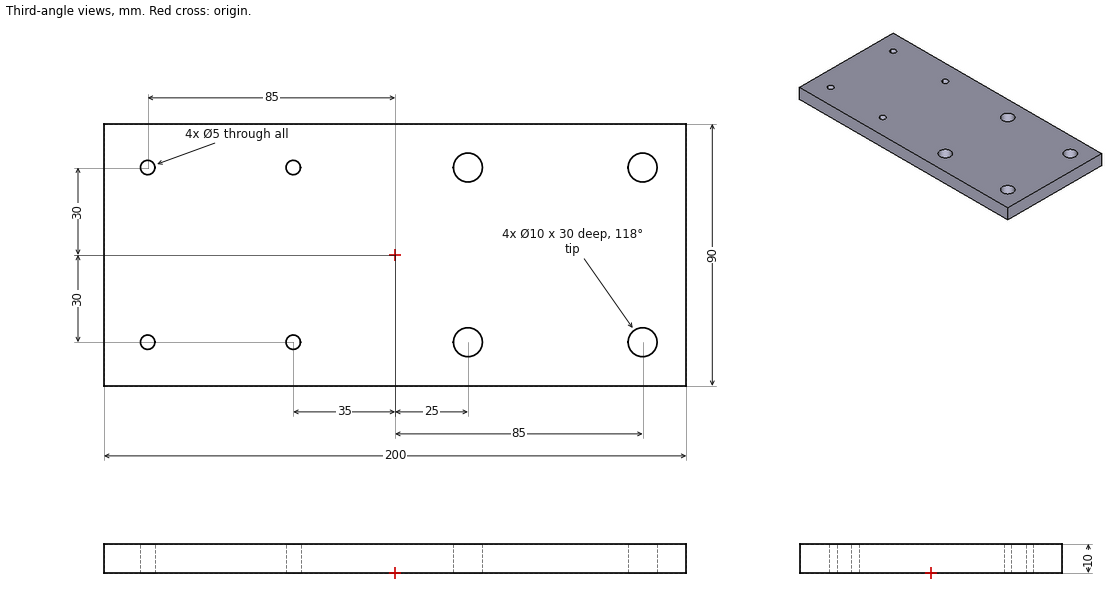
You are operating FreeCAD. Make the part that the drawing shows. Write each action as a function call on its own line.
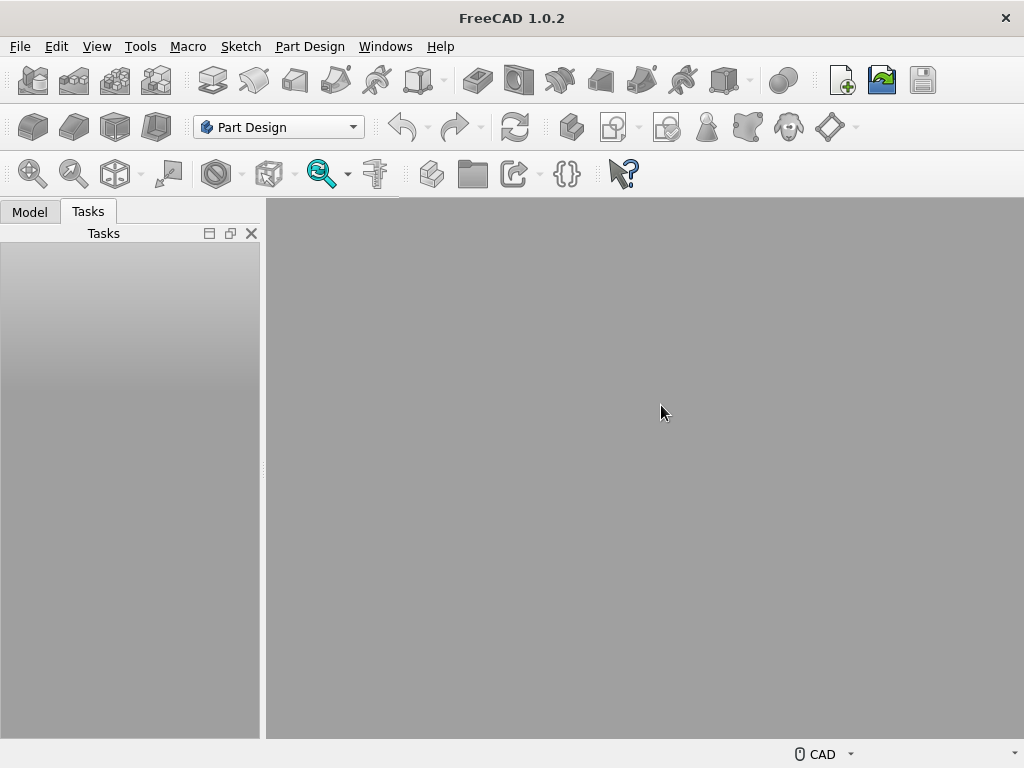
key(ctrl+n)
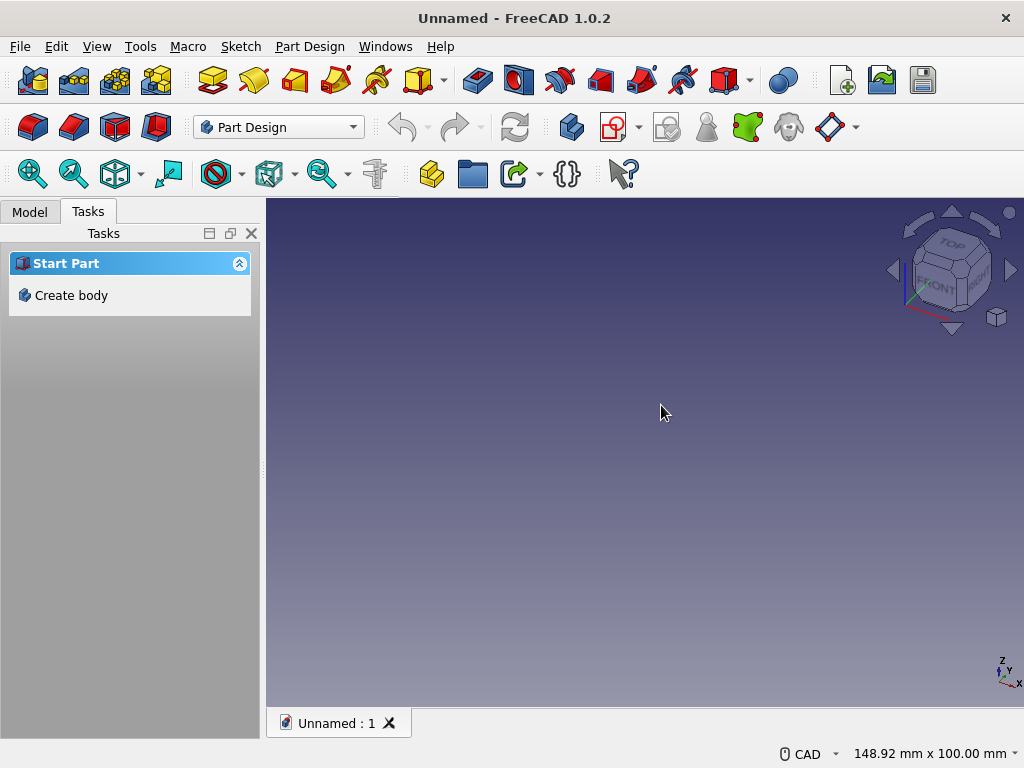
click(612, 128)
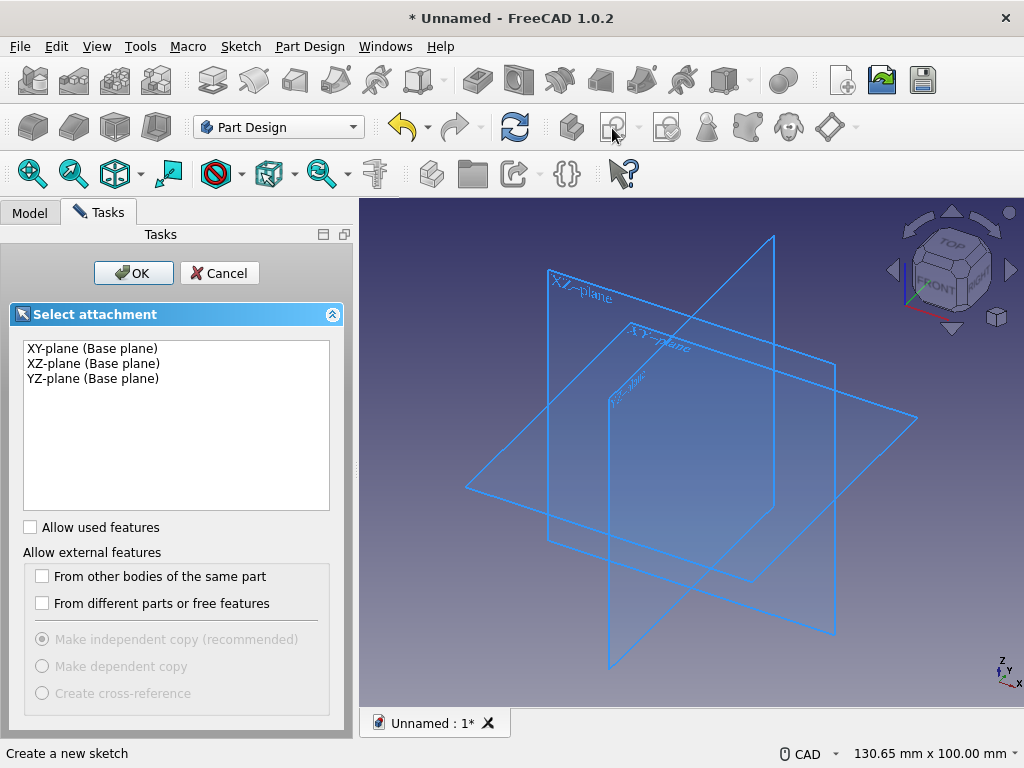
click(84, 348)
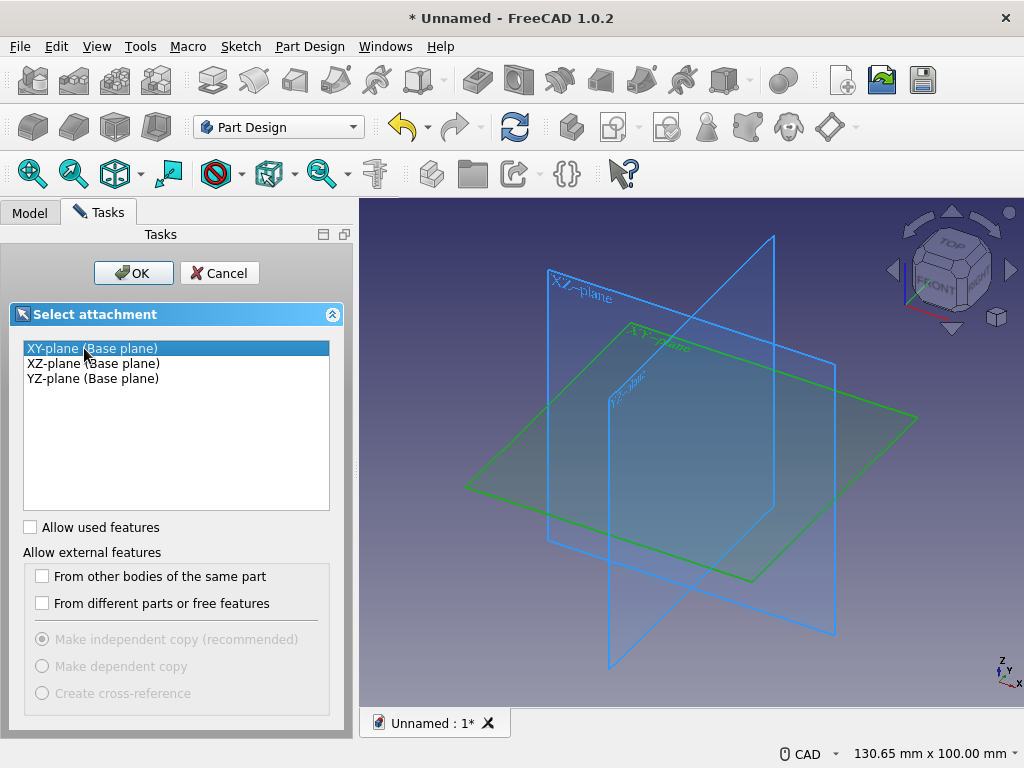
click(134, 273)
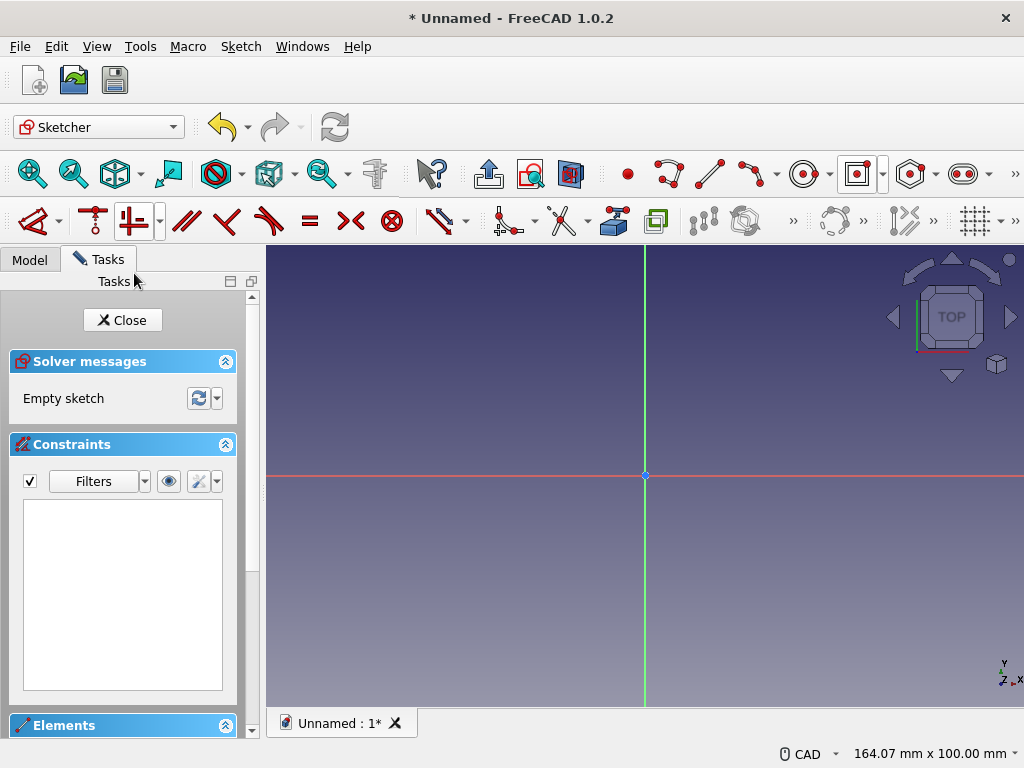
scroll(521, 476, down, 4)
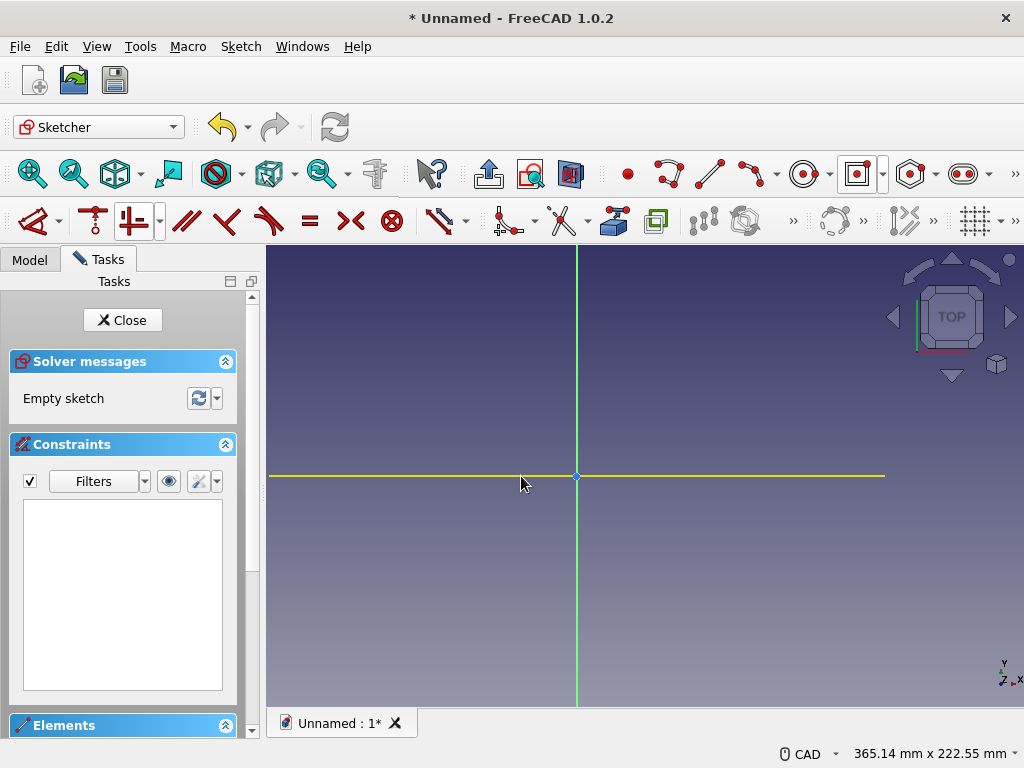
click(856, 174)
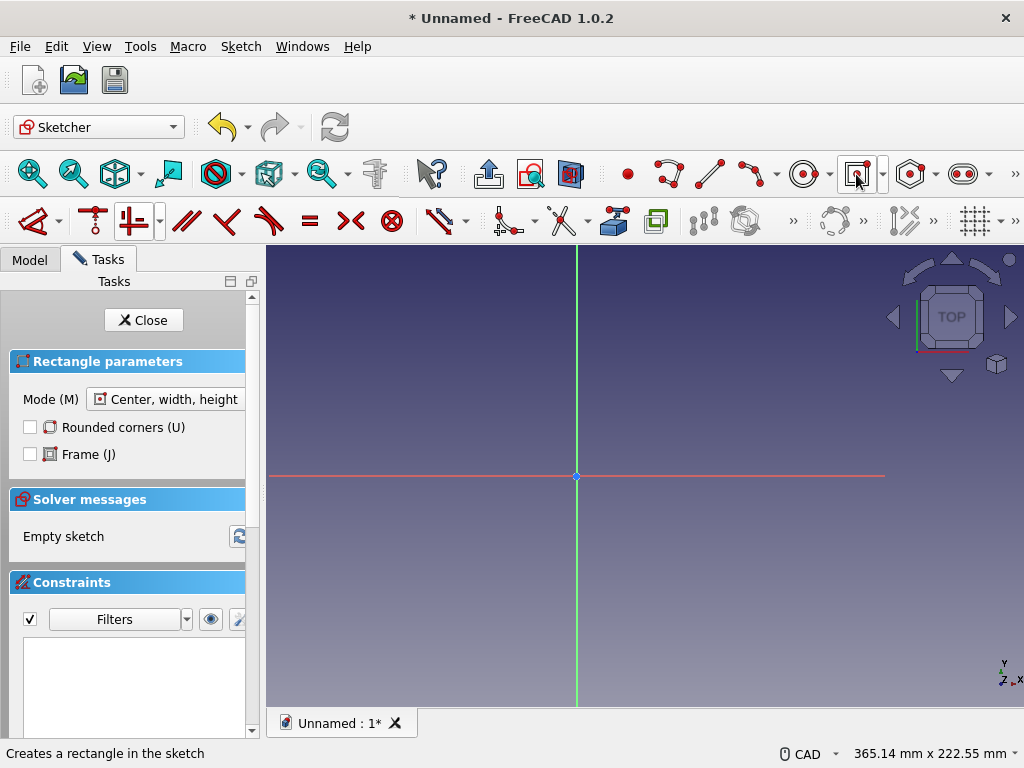
click(577, 476)
move(784, 383)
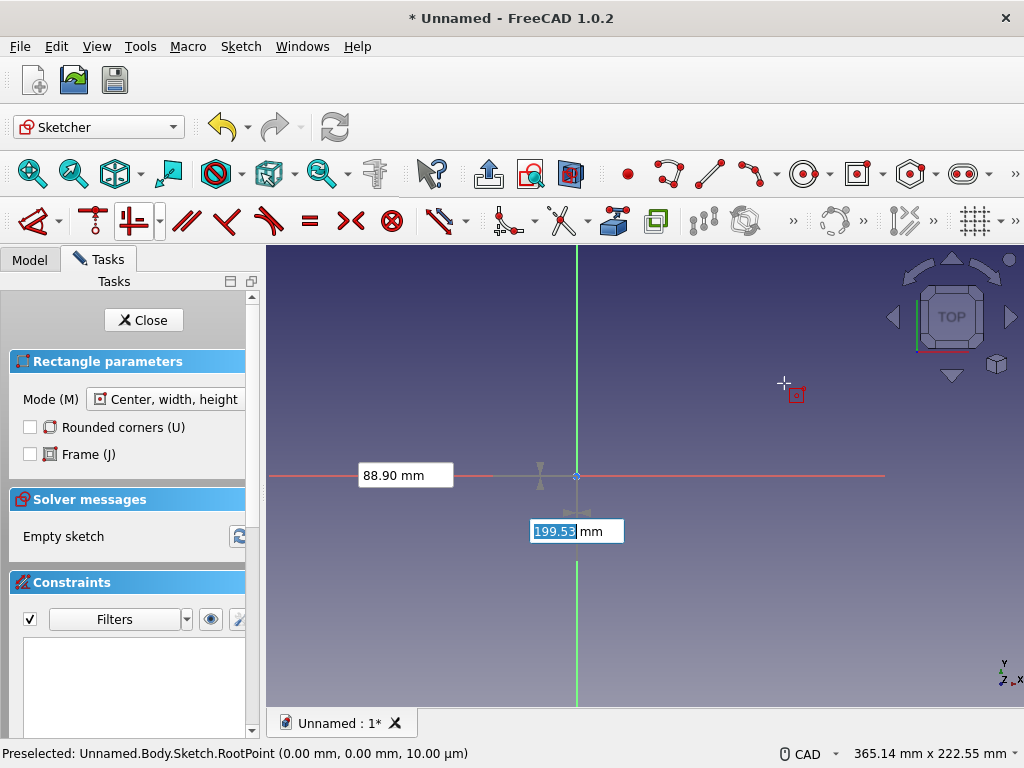
text(200)
key(Tab)
text(90)
key(Return)
key(Escape)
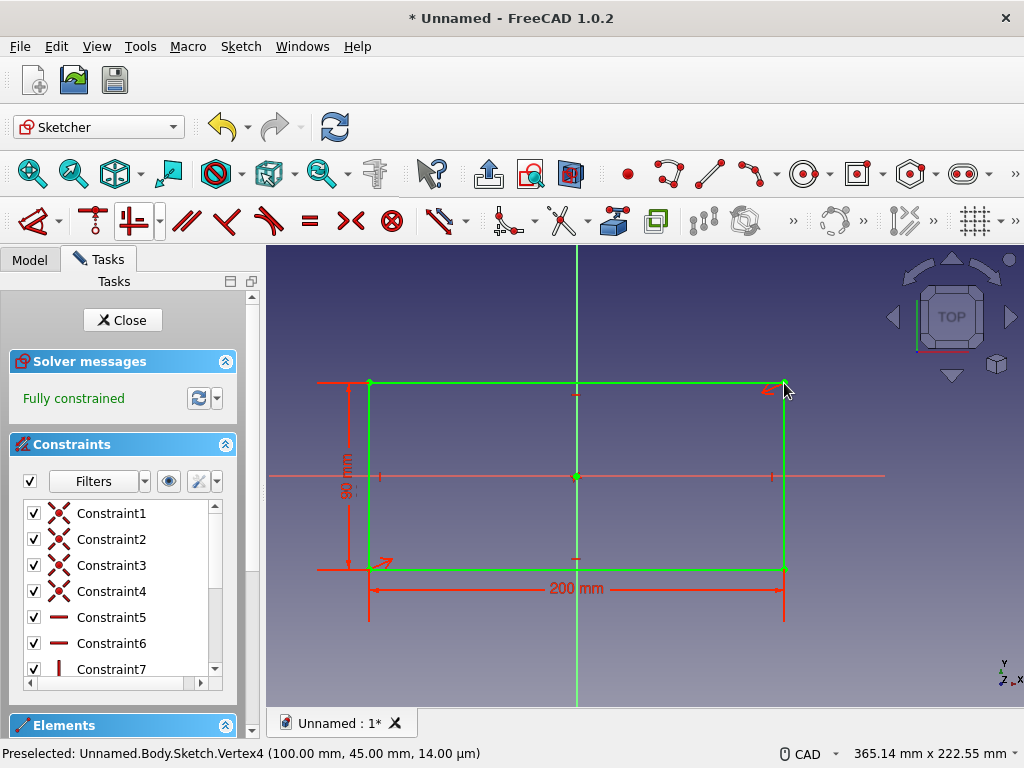
click(123, 320)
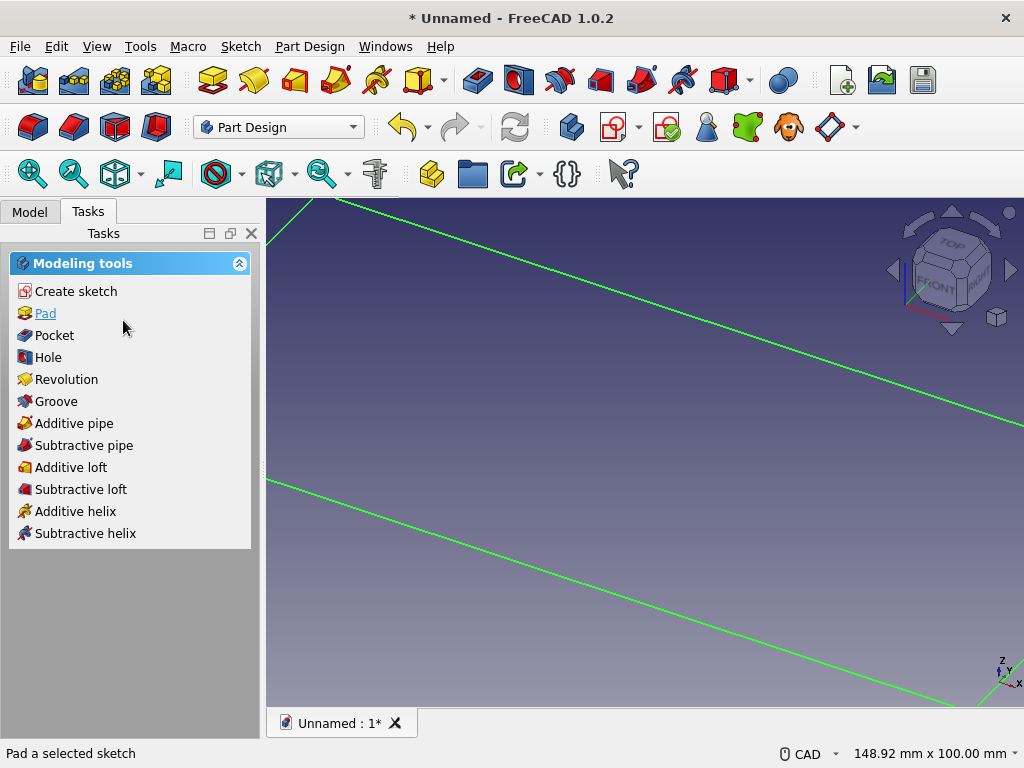
click(213, 80)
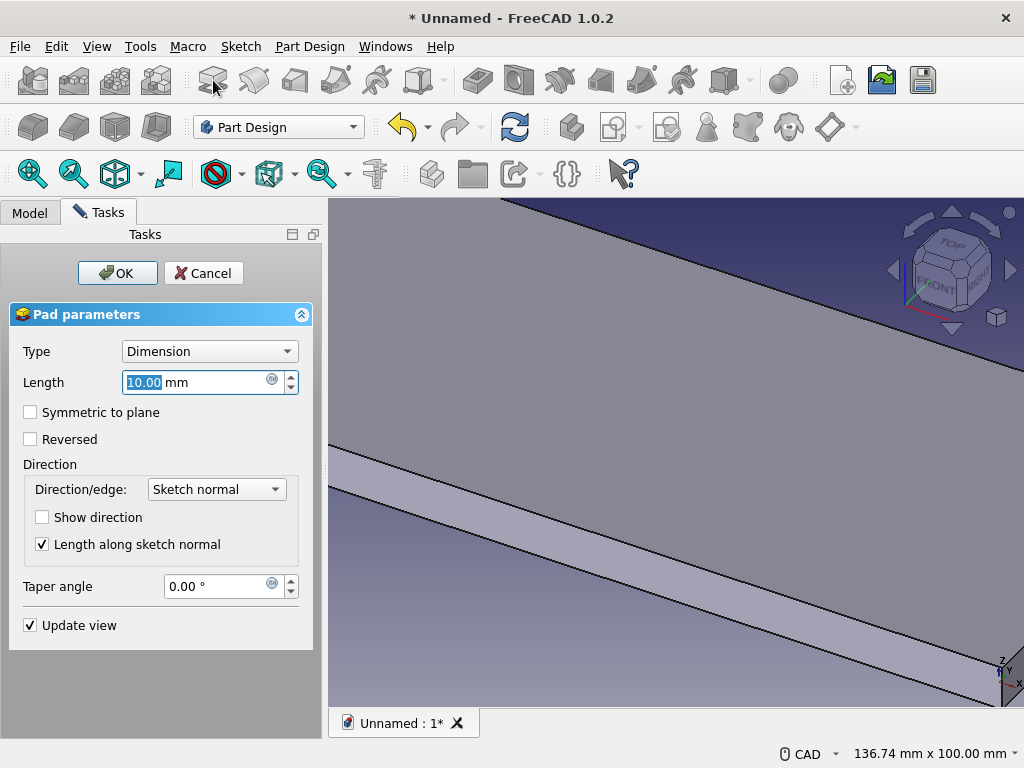
text(10)
key(Tab)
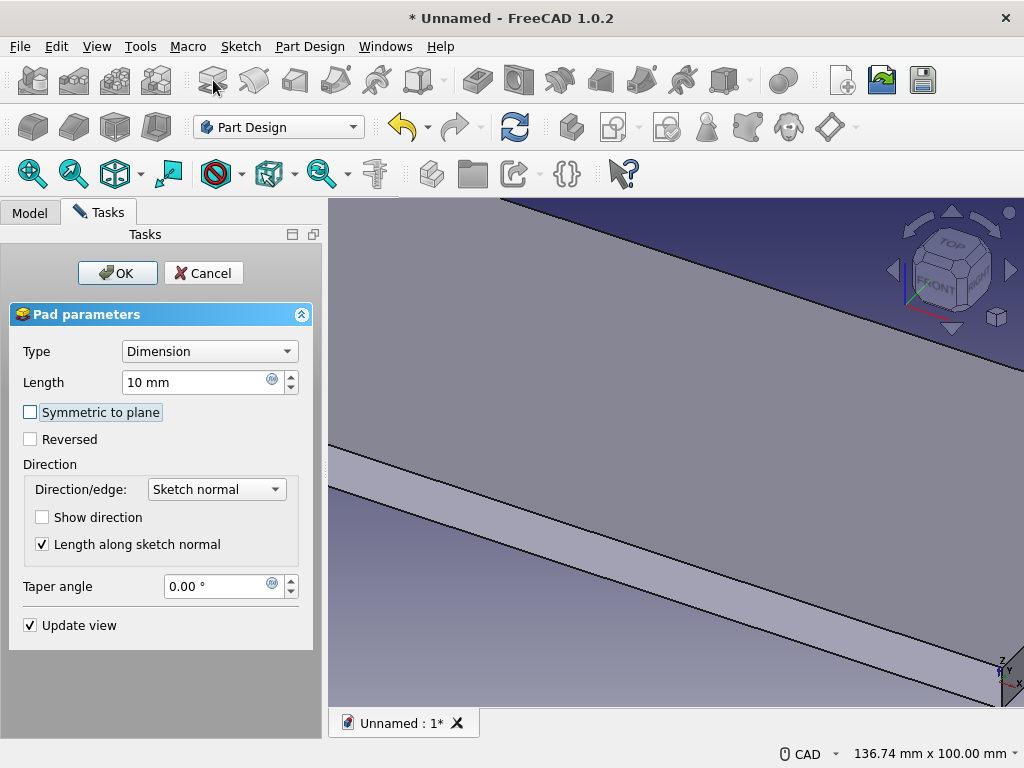
click(118, 273)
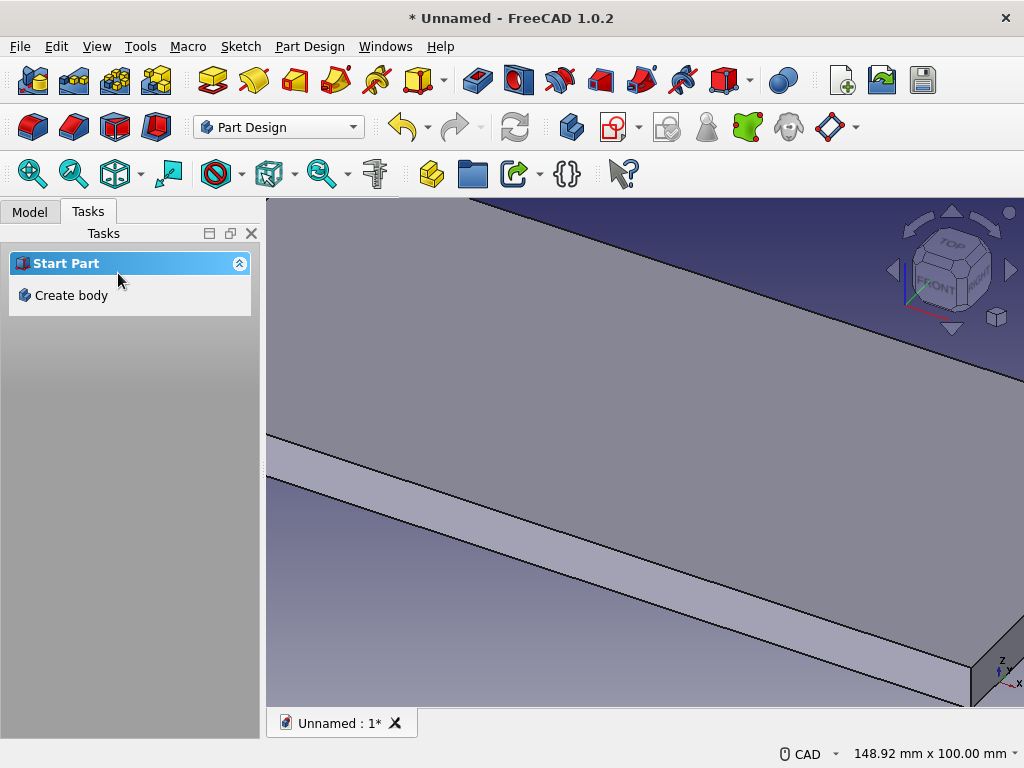
click(33, 174)